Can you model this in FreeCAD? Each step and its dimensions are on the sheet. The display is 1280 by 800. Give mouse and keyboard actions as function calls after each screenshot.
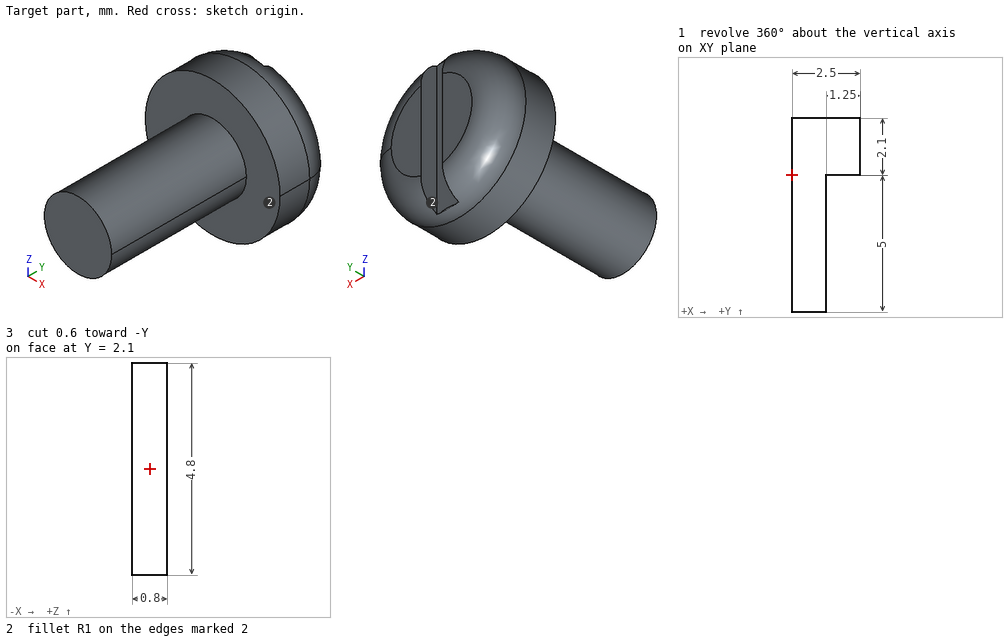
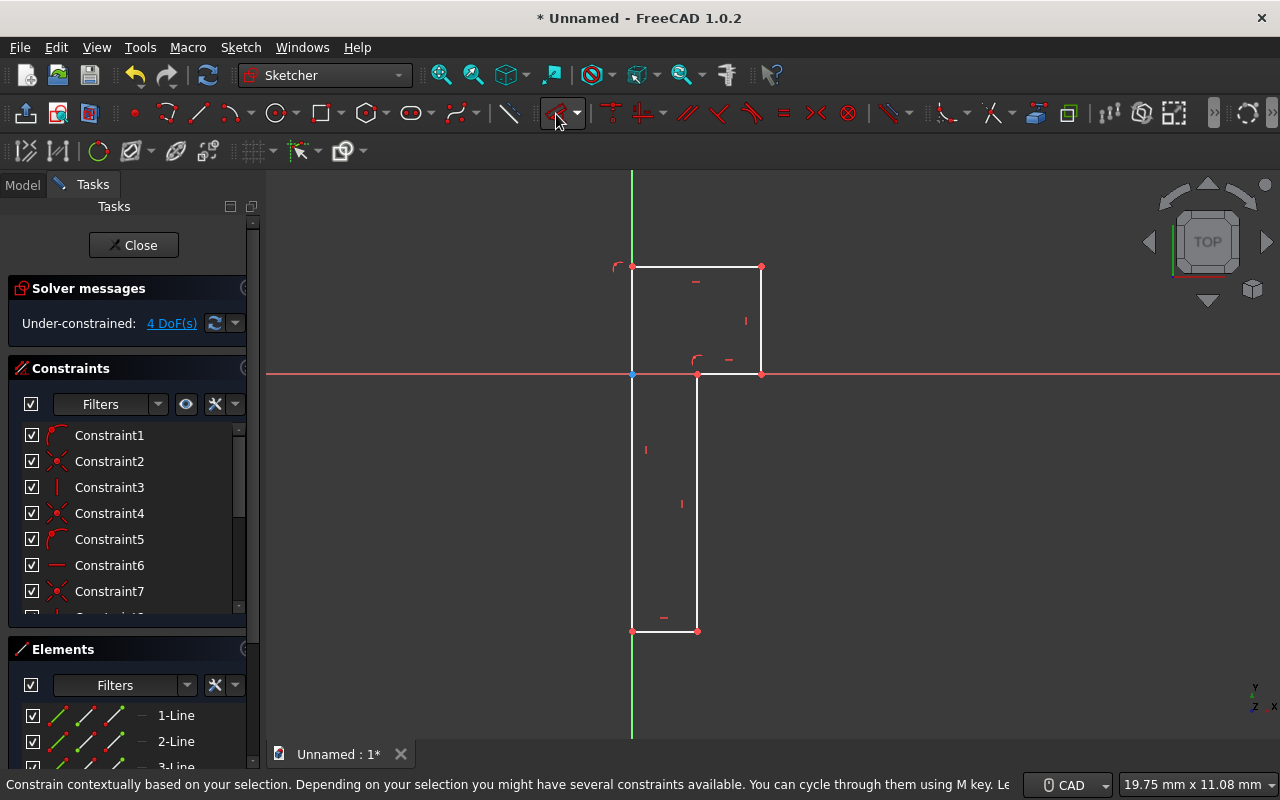
click(697, 555)
click(731, 503)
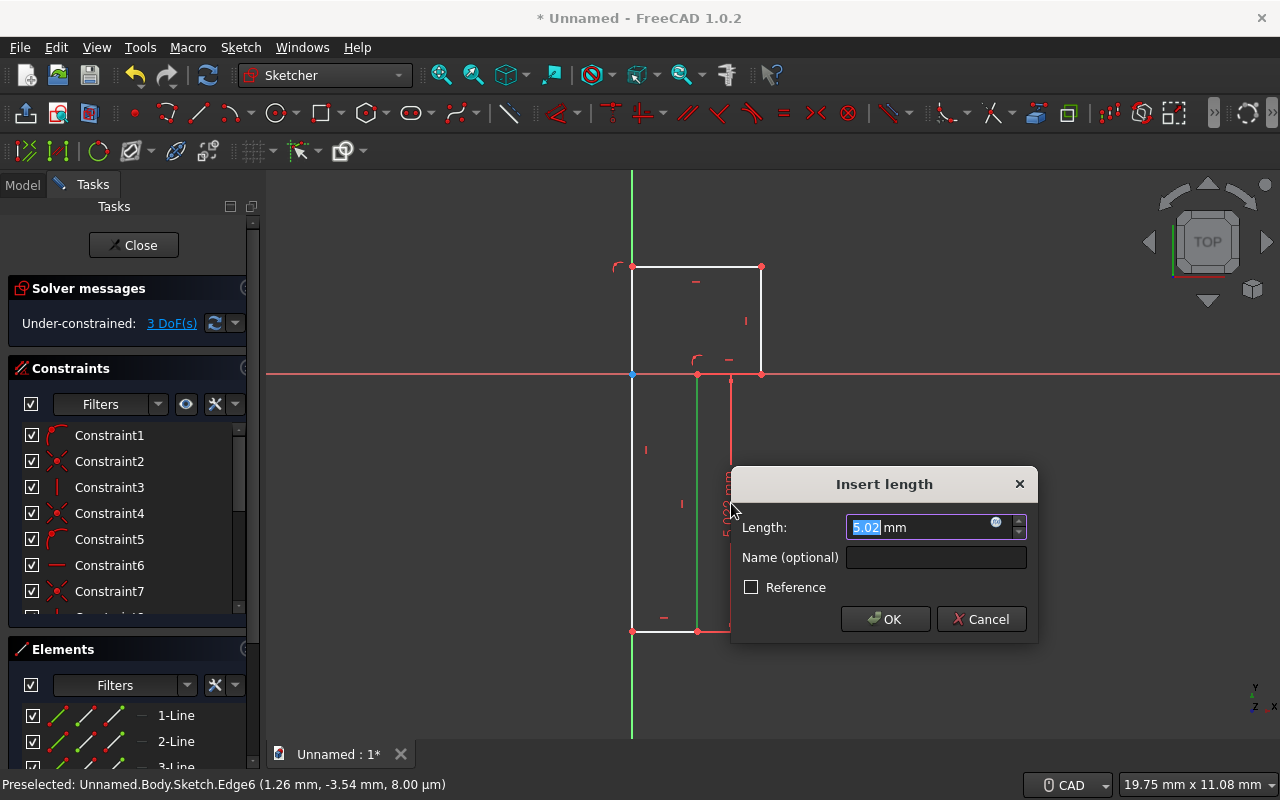
text(5)
key(Return)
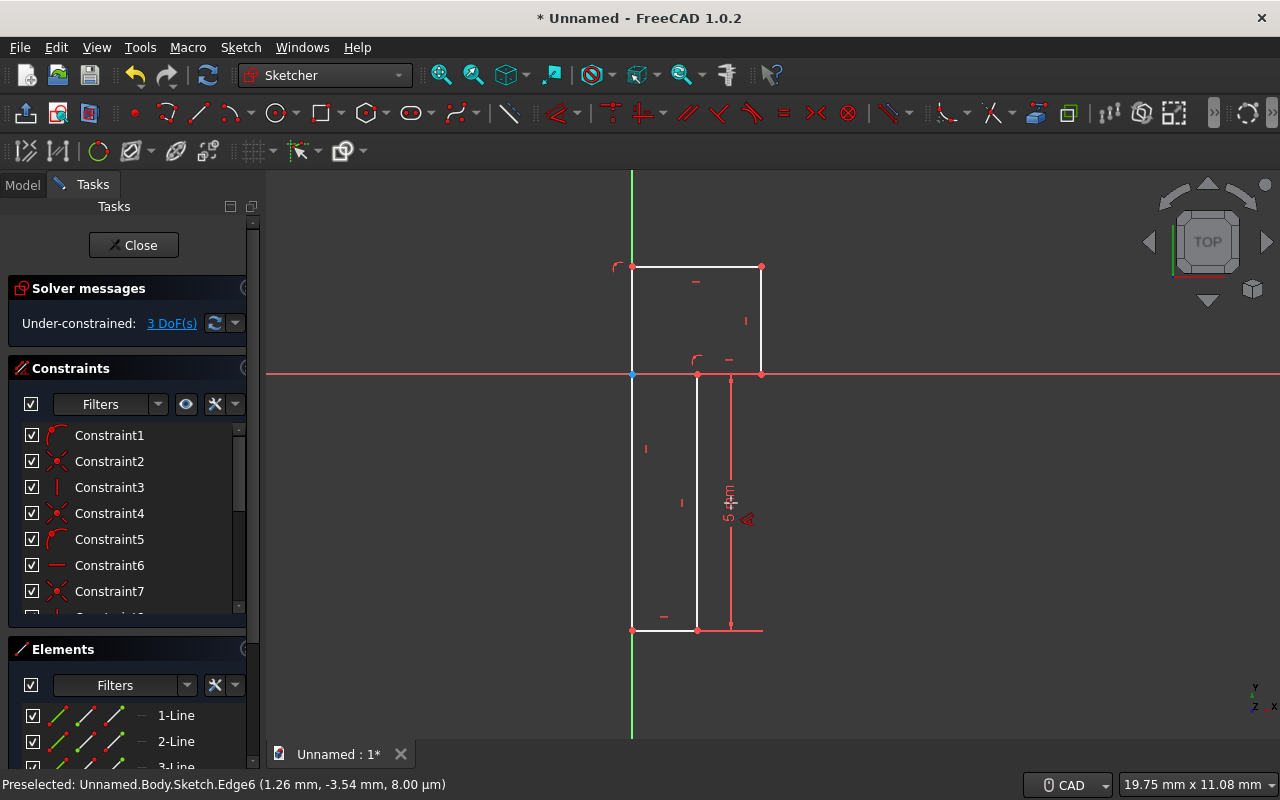
click(761, 342)
click(795, 321)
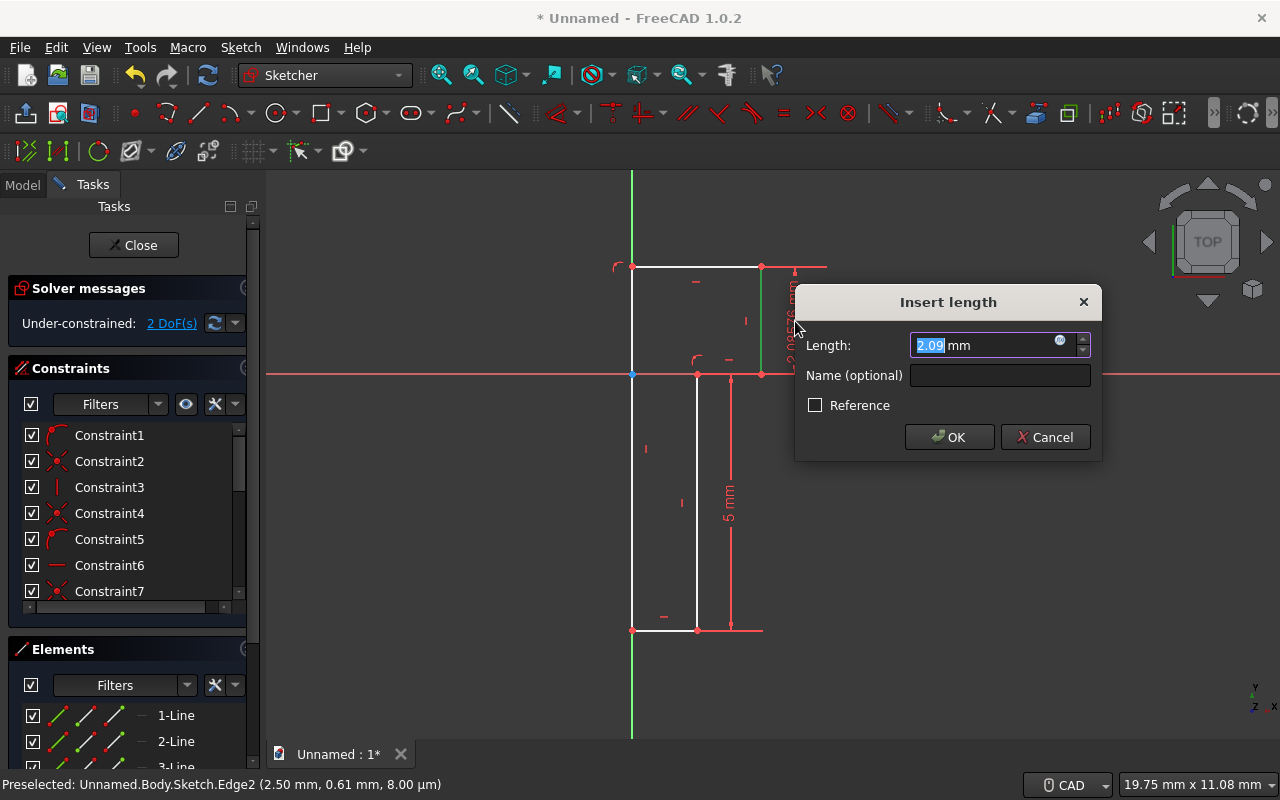
text(2.1)
key(Return)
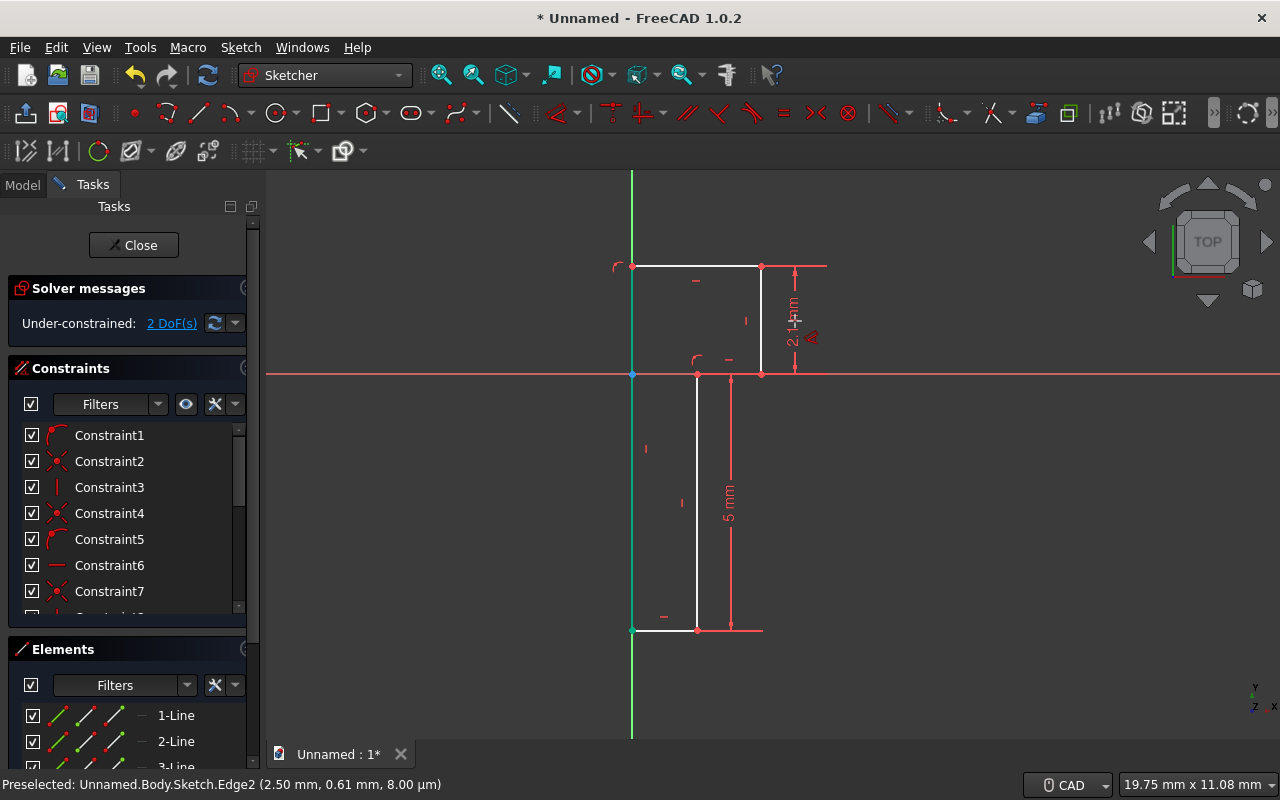
click(722, 266)
click(697, 232)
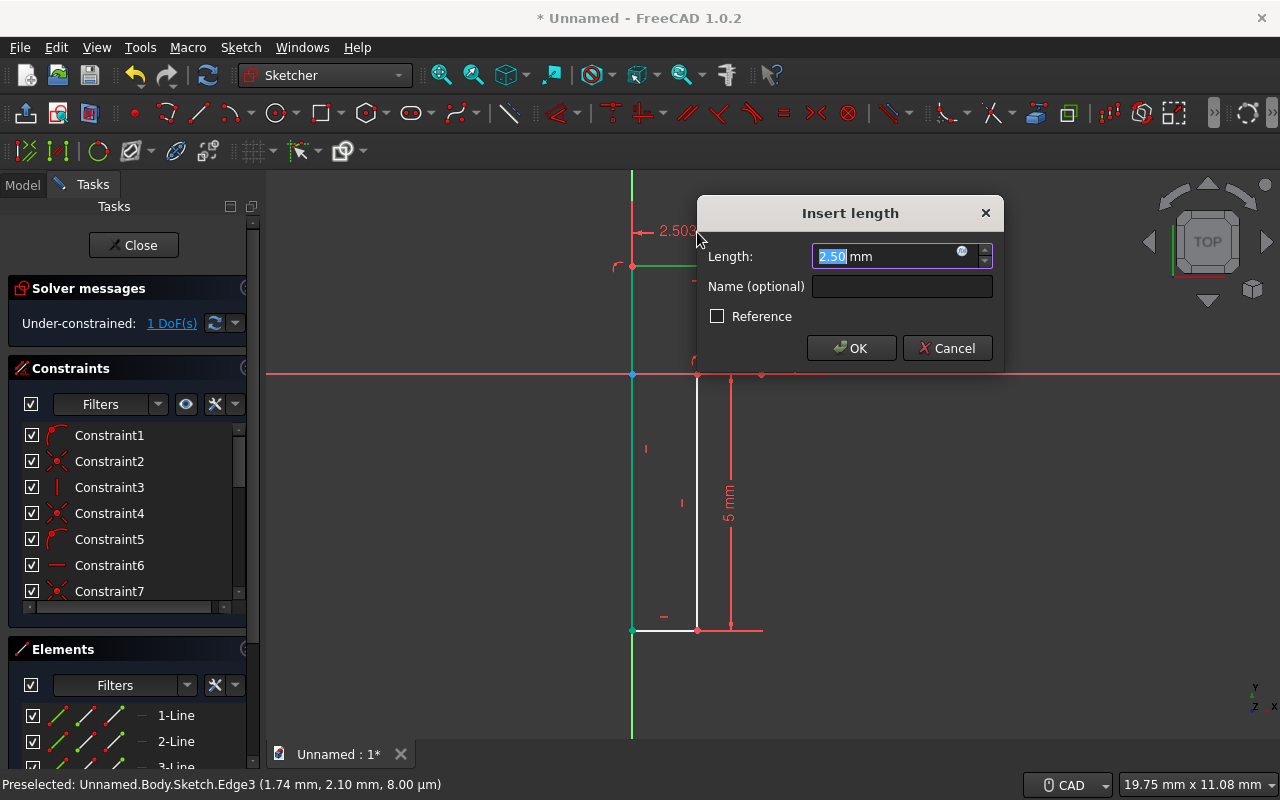
text(2.5)
key(Return)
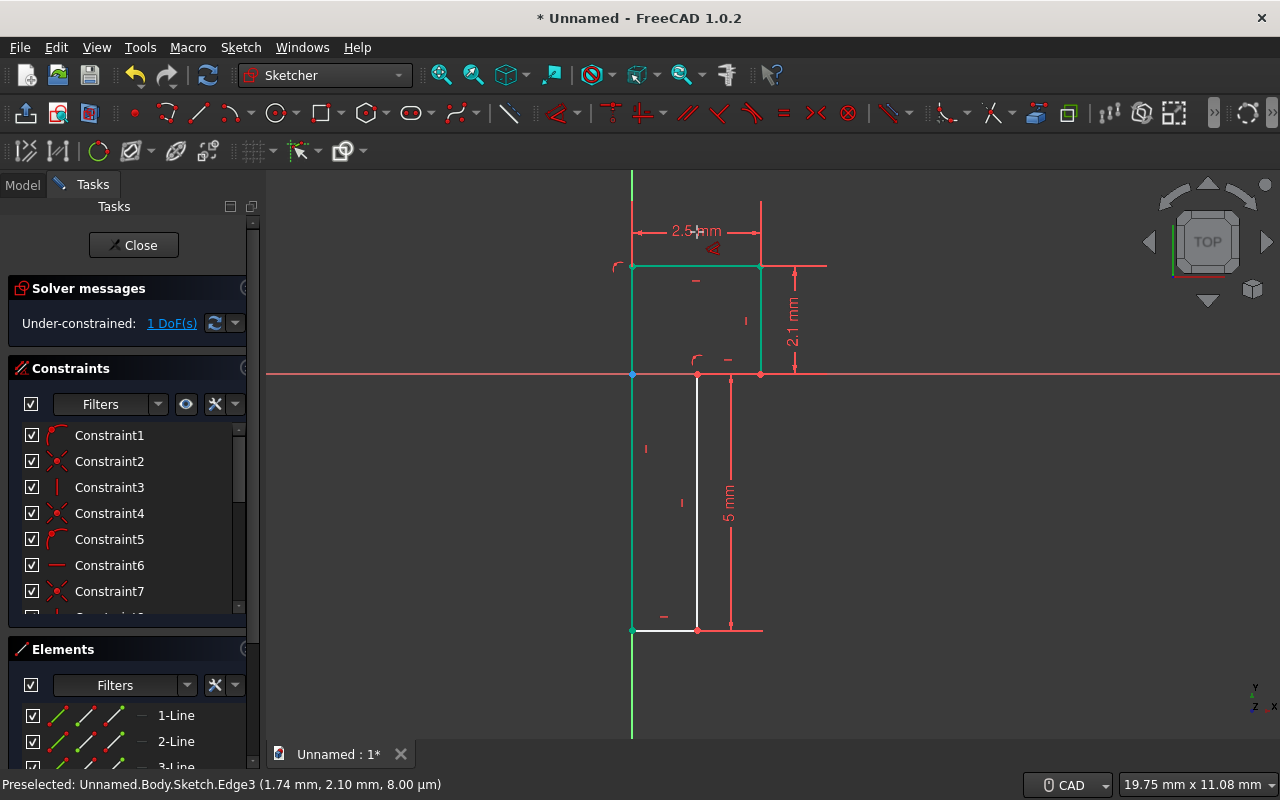
click(716, 374)
click(714, 340)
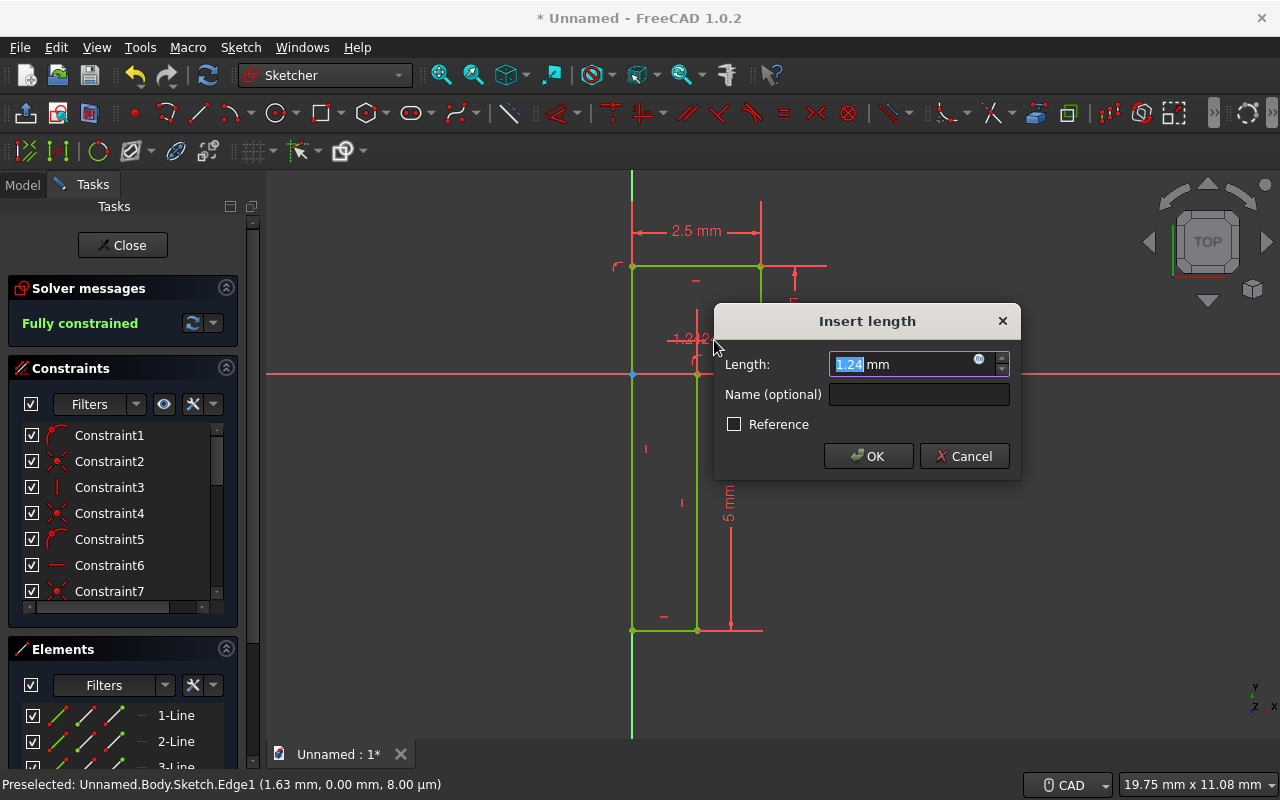
text(1.25)
key(Return)
key(Escape)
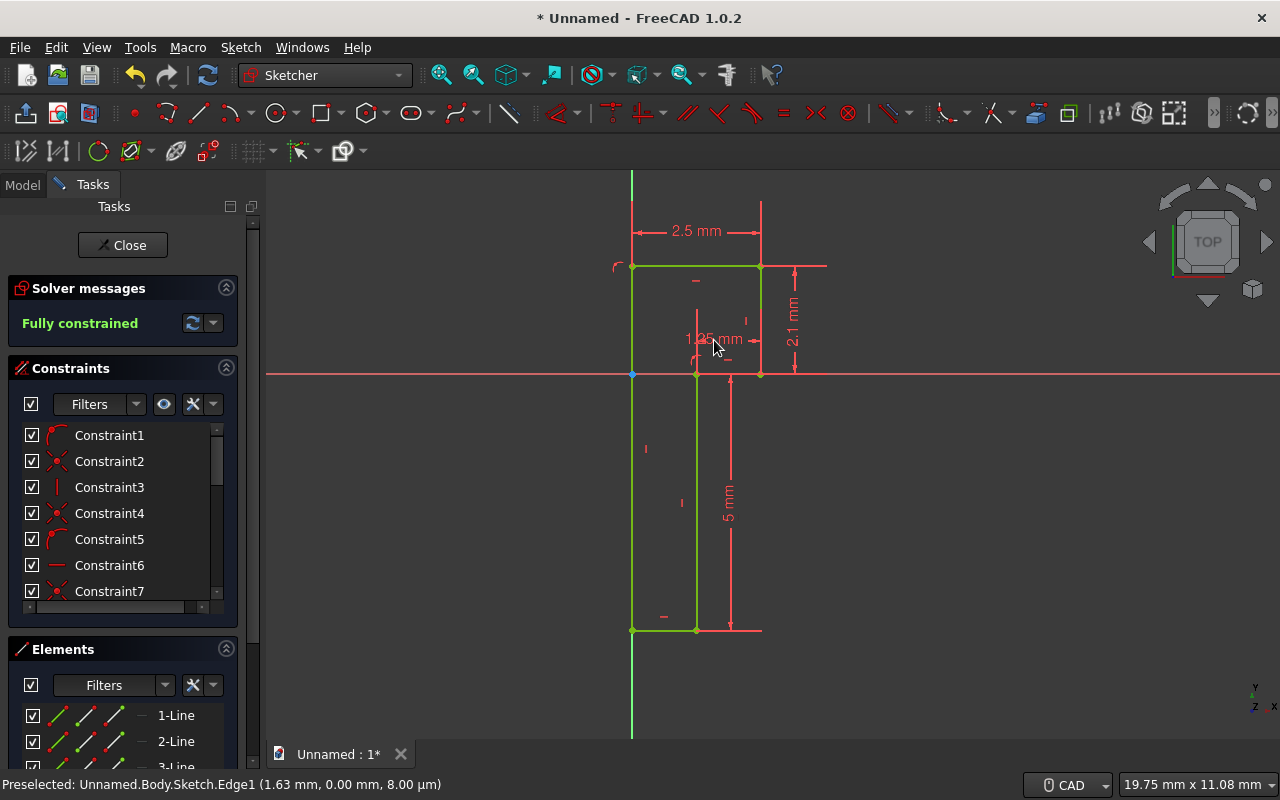
click(123, 245)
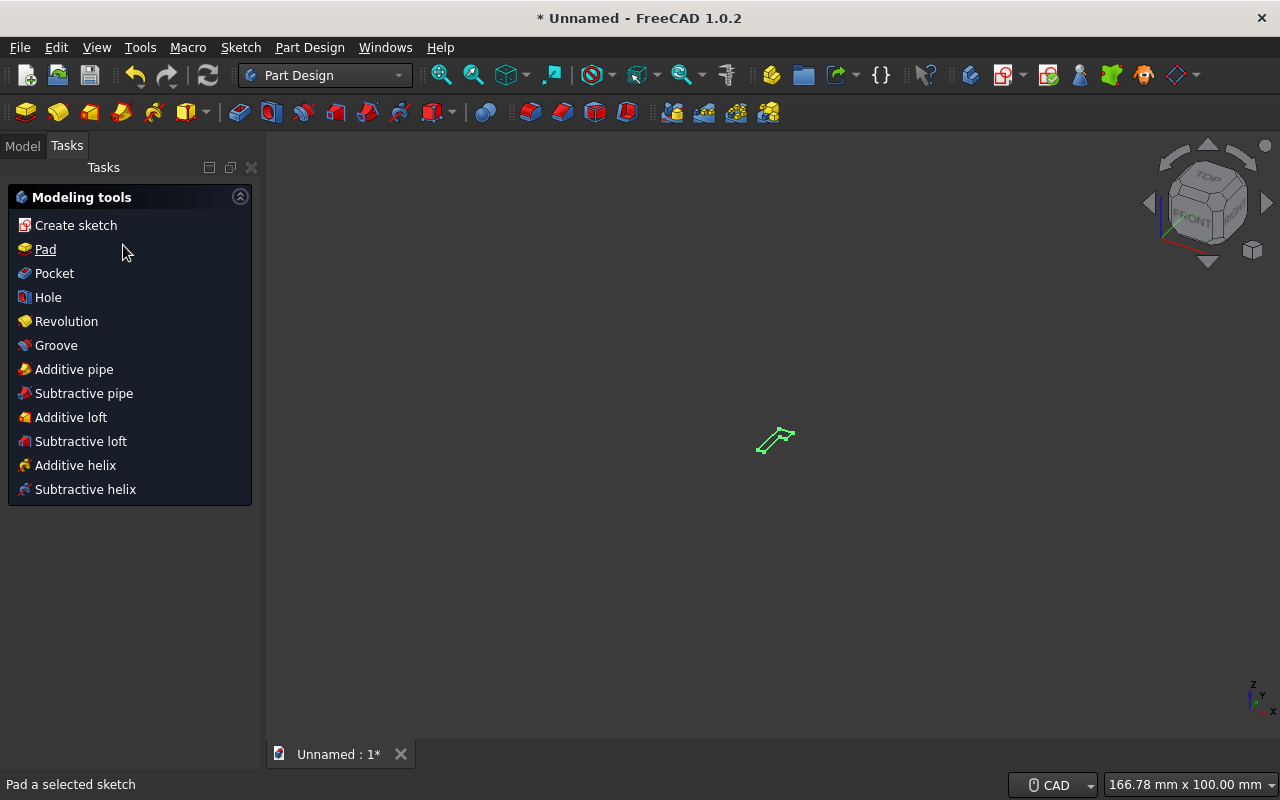
click(58, 112)